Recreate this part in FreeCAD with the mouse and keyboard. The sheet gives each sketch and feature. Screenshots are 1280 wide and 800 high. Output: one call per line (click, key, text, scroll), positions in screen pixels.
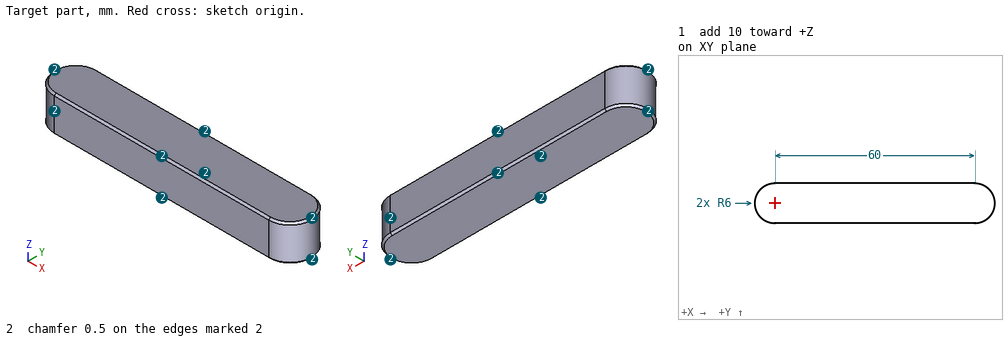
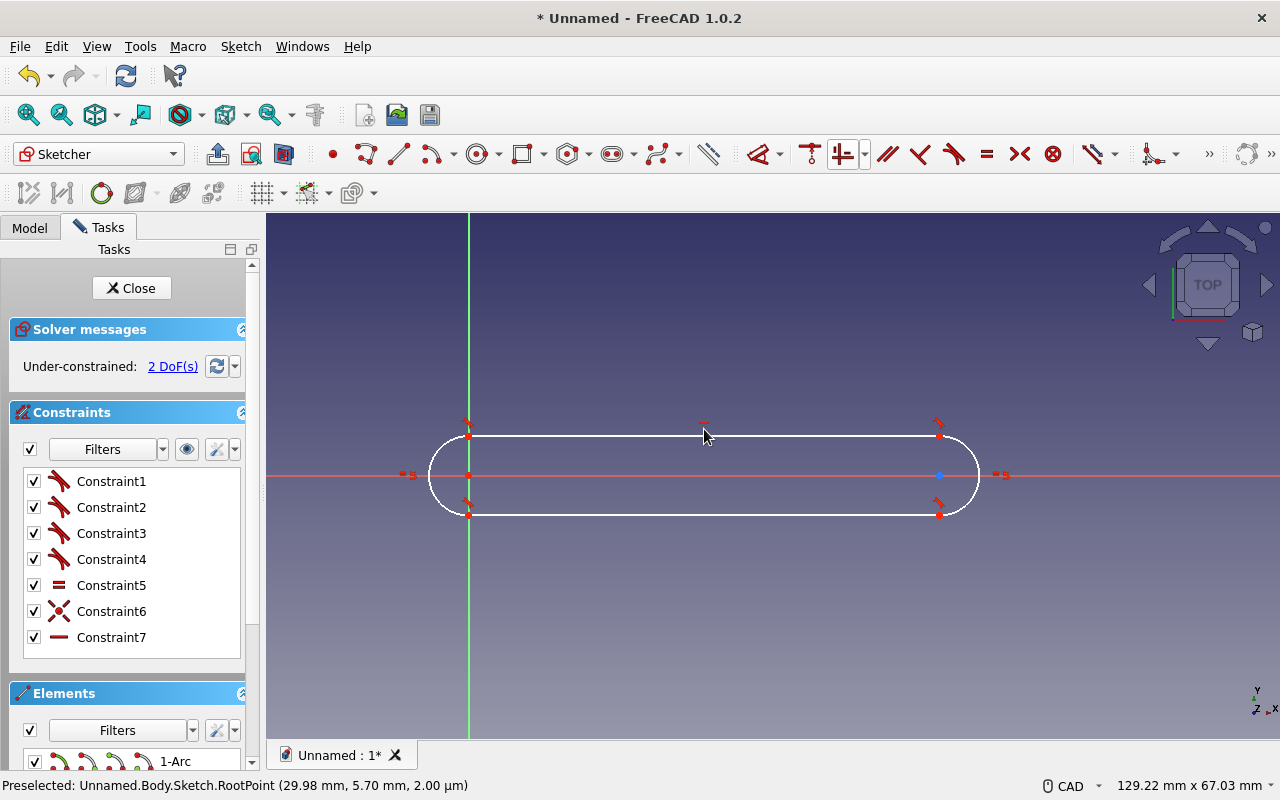
click(437, 452)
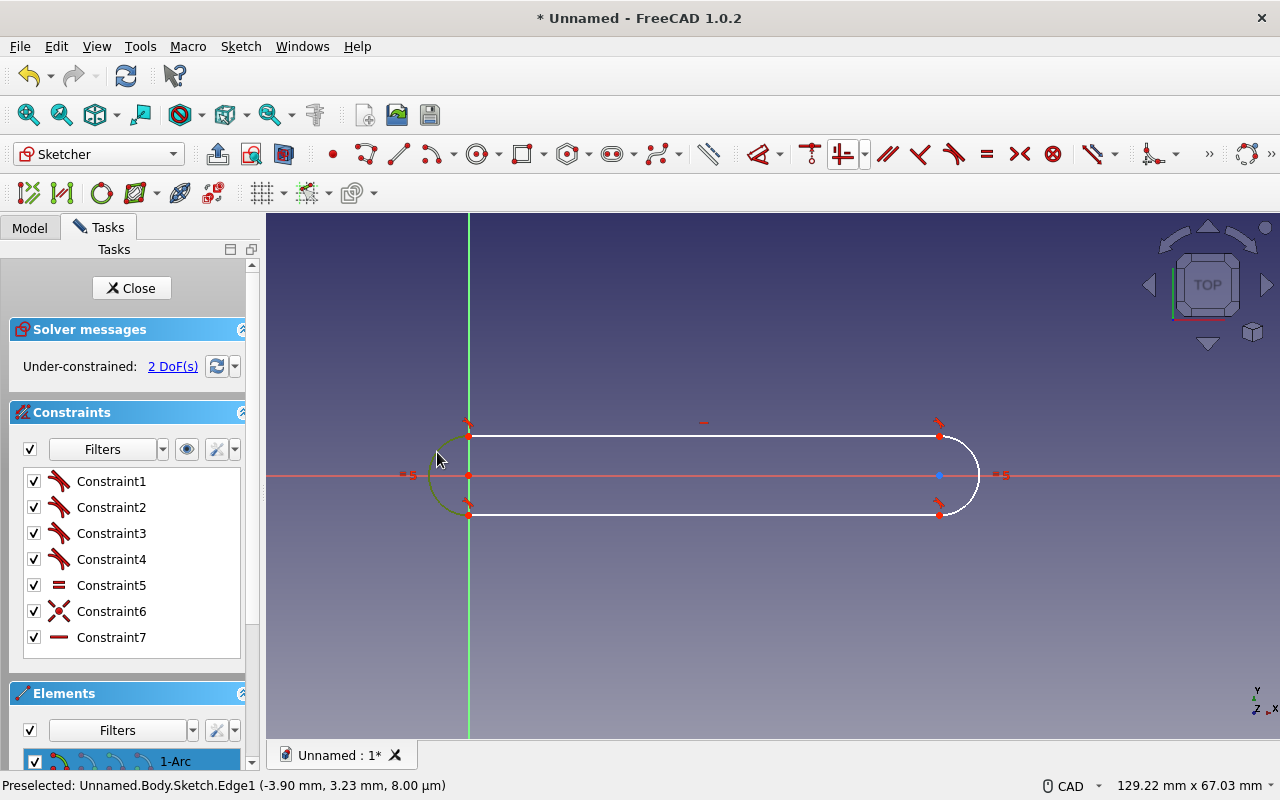
click(780, 154)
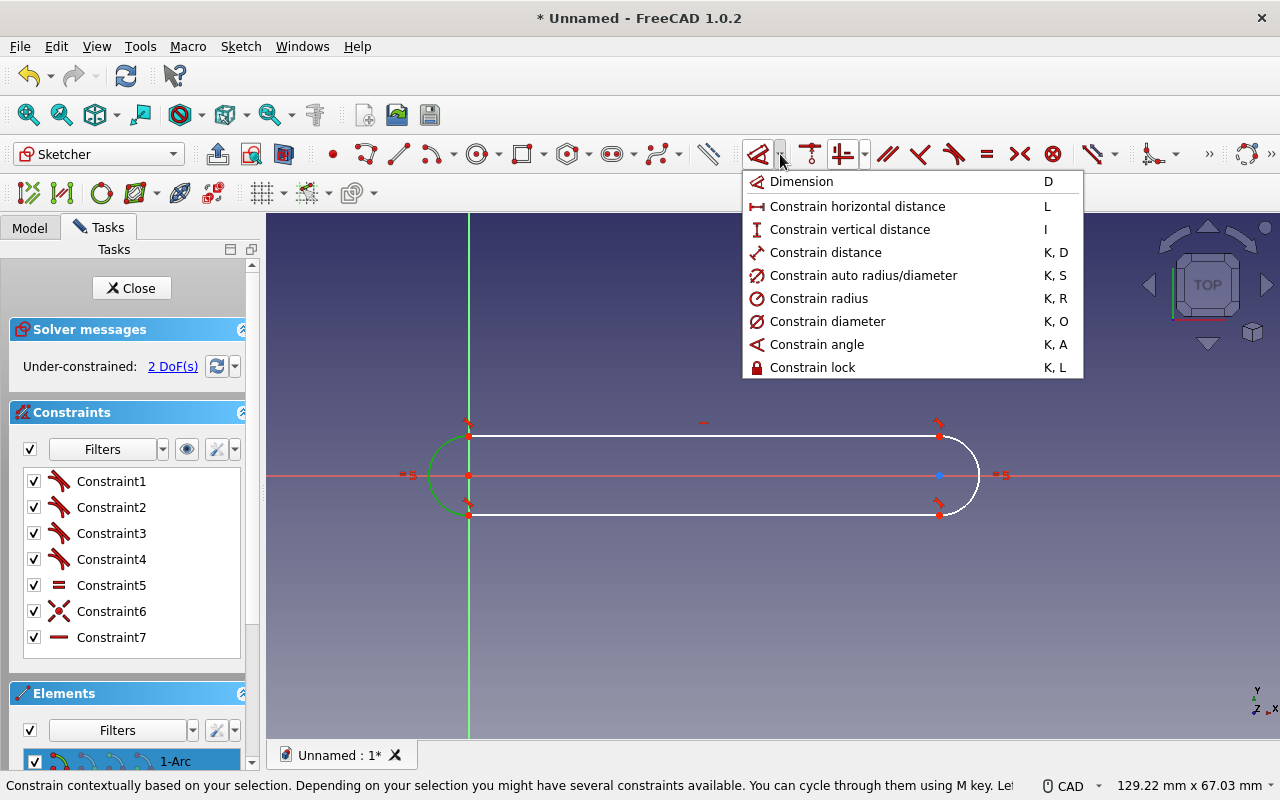
click(913, 298)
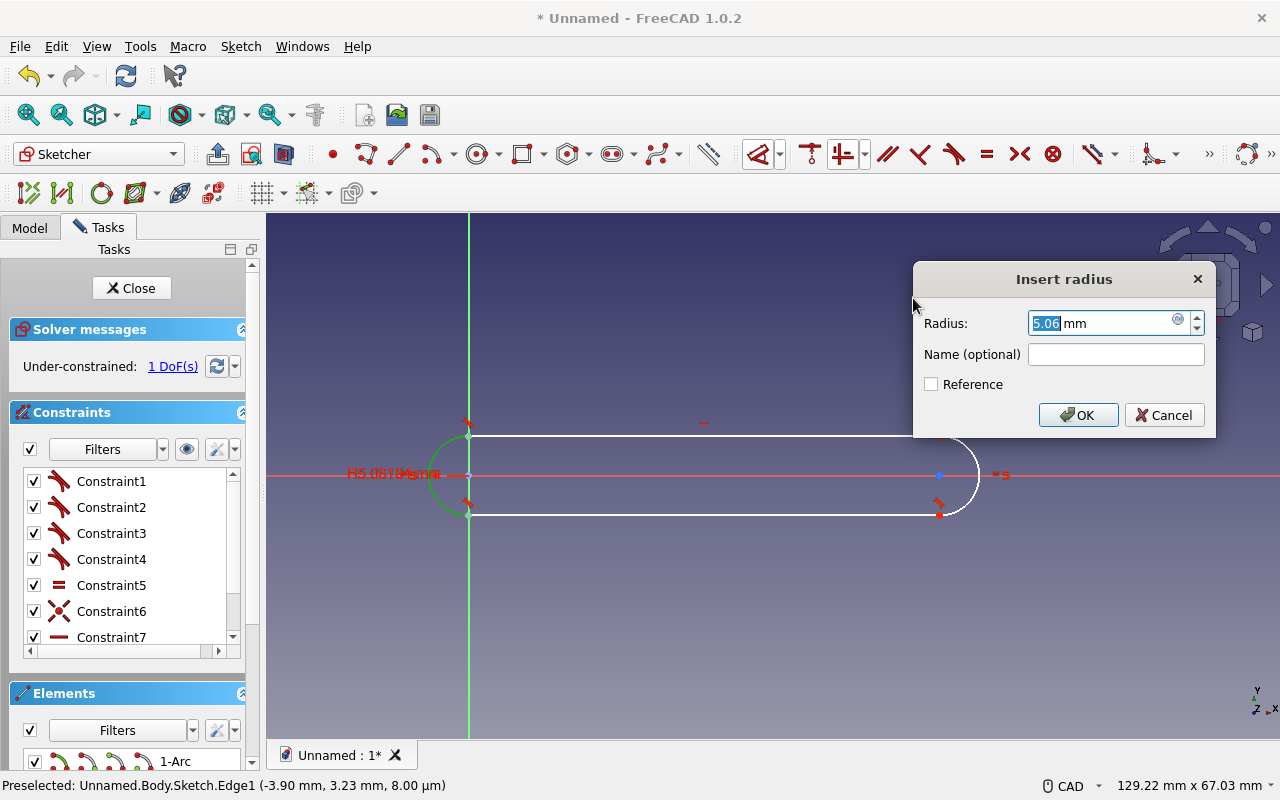
text(6)
key(Return)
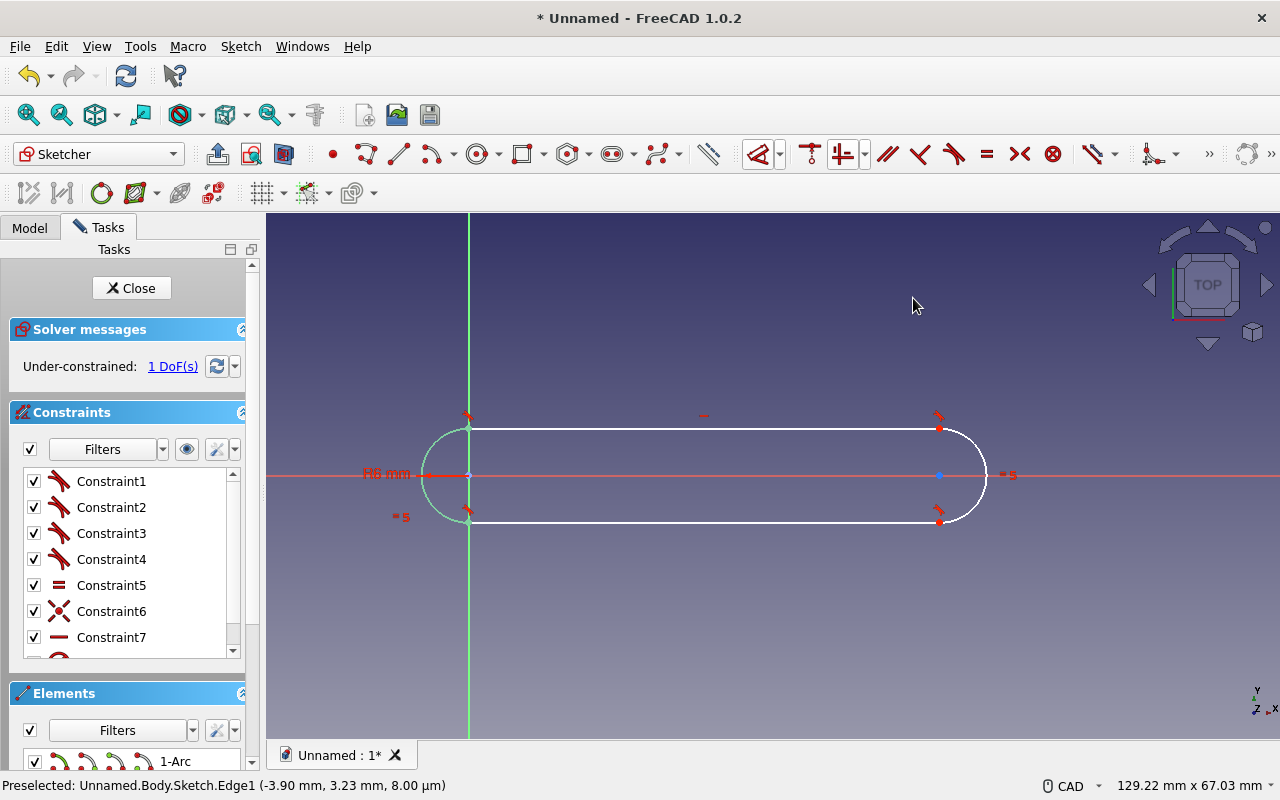
click(610, 429)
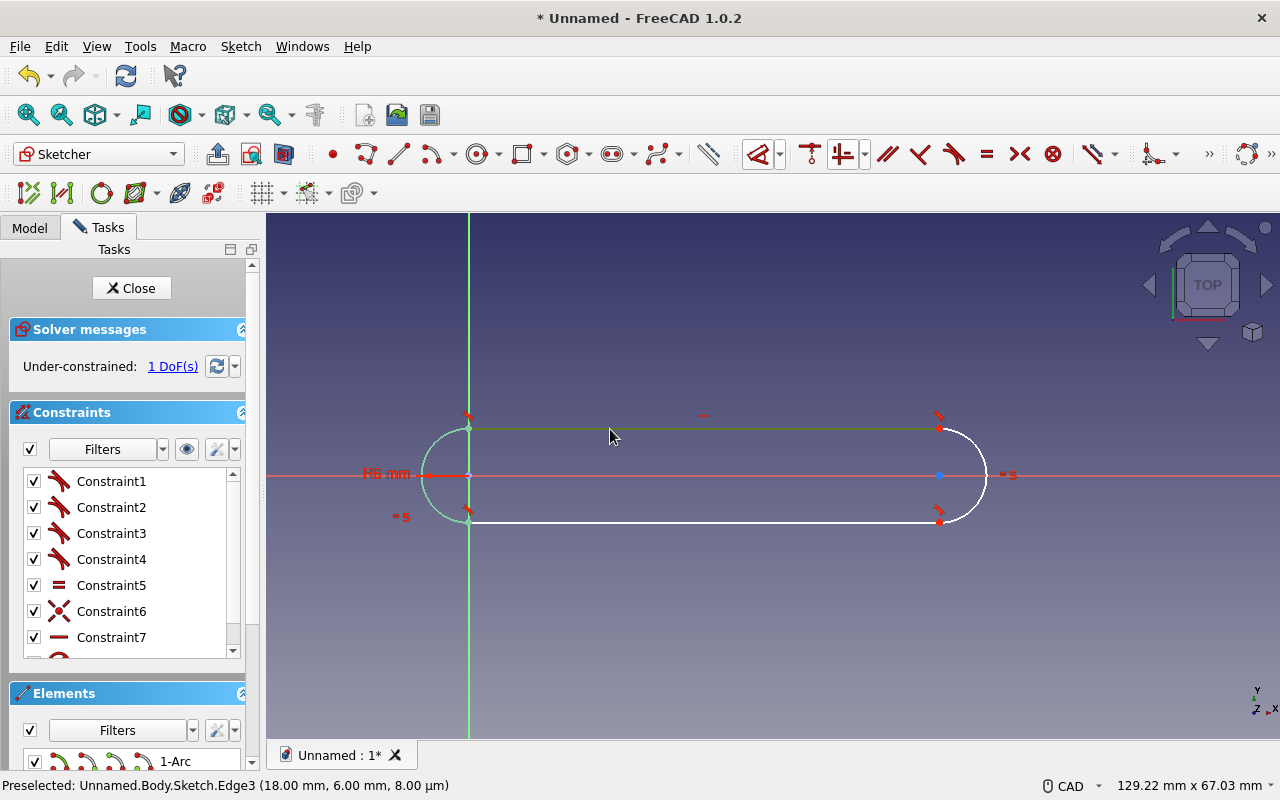
click(780, 154)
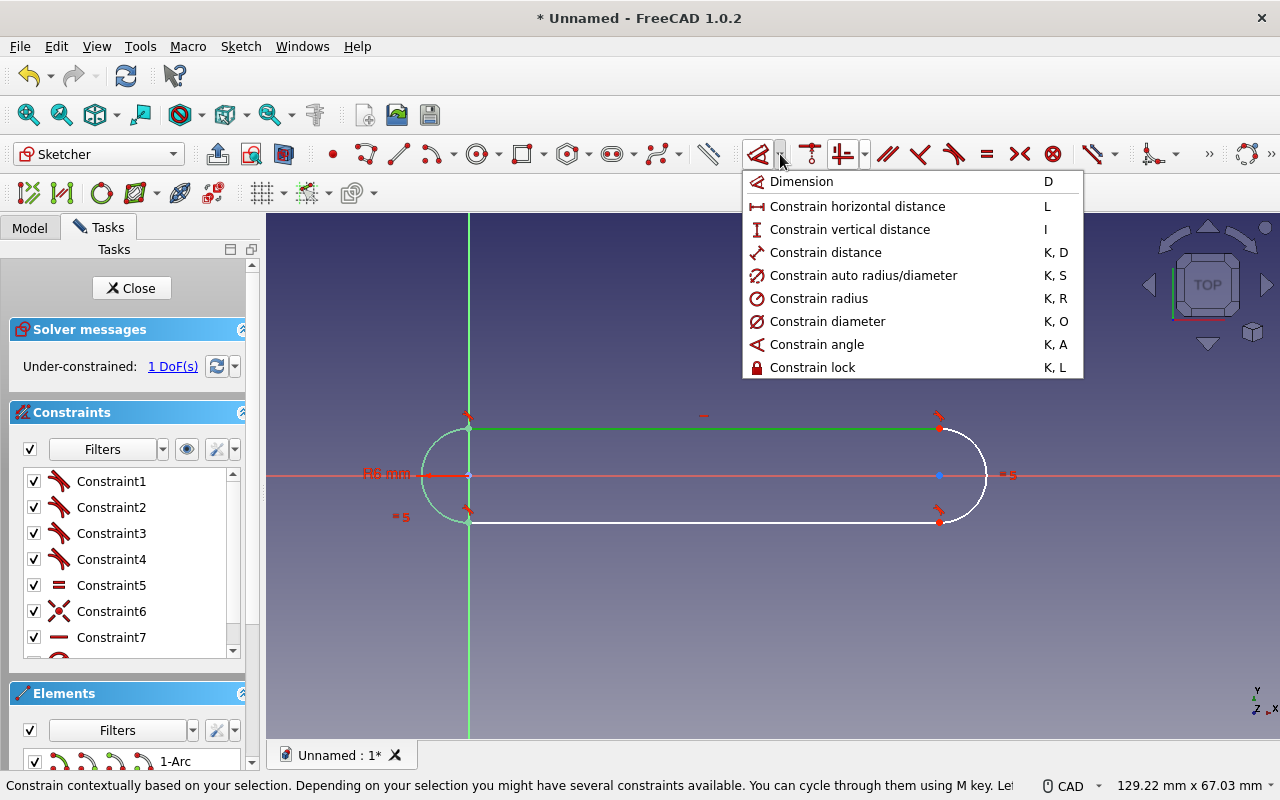
click(913, 206)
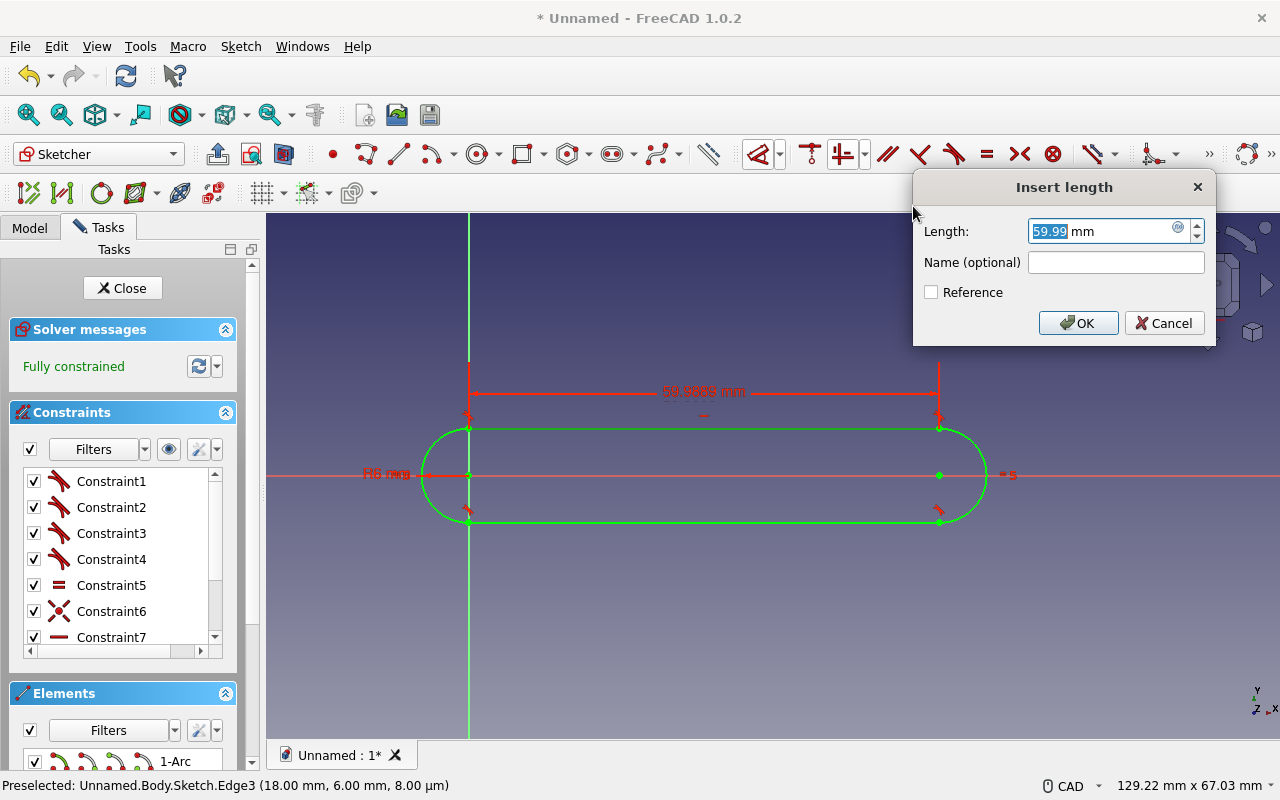
text(60)
key(Return)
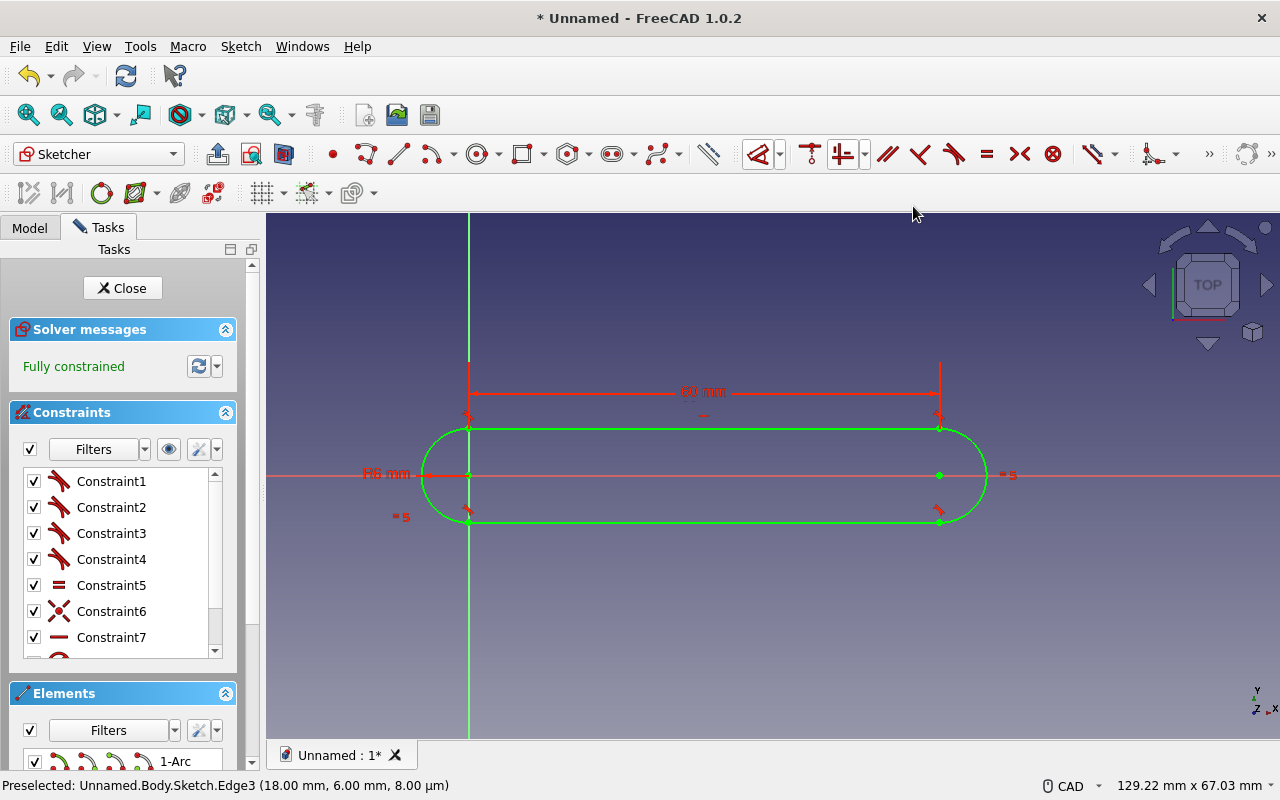
click(123, 288)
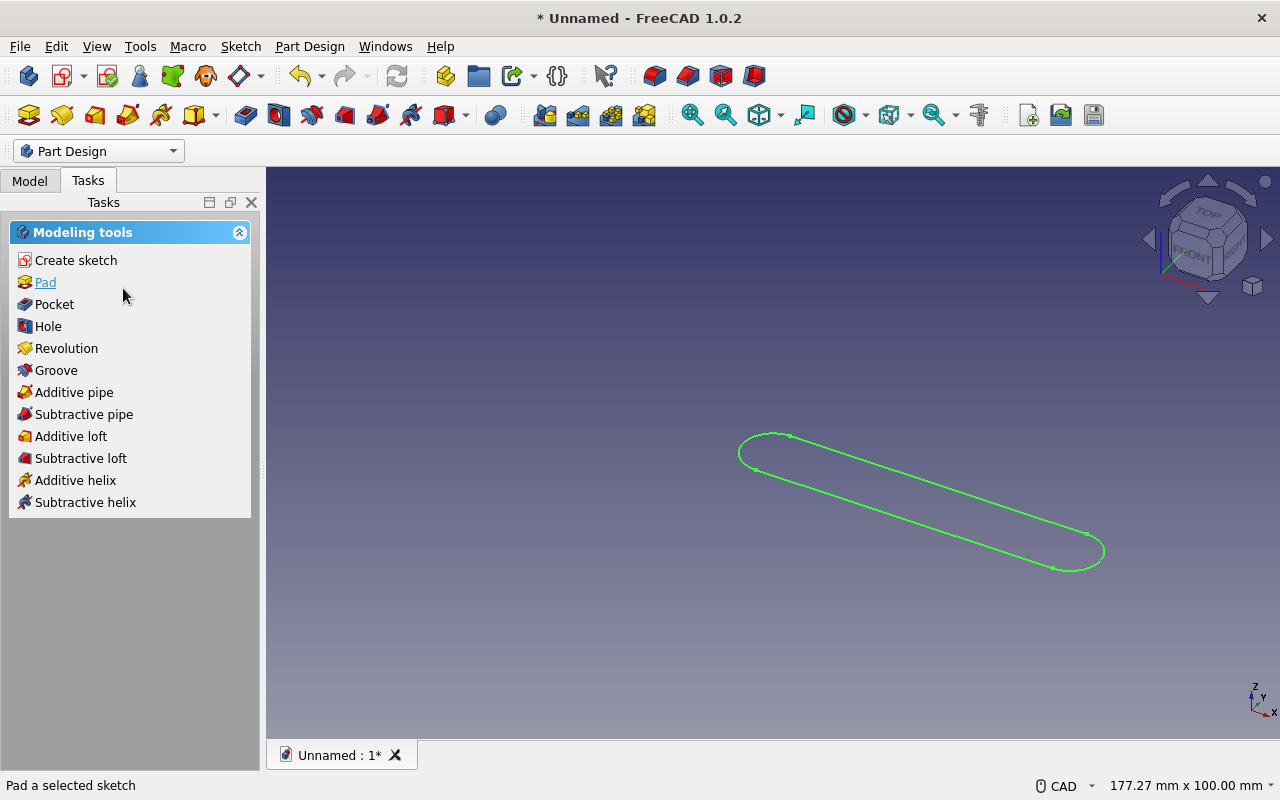
click(29, 116)